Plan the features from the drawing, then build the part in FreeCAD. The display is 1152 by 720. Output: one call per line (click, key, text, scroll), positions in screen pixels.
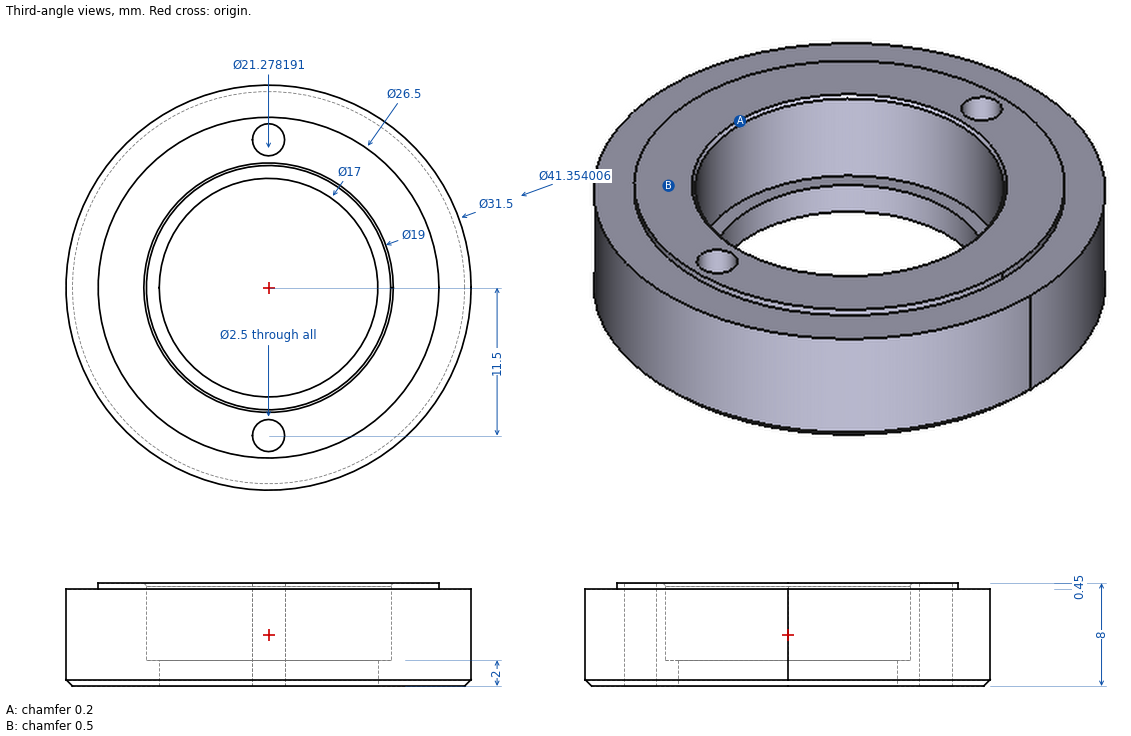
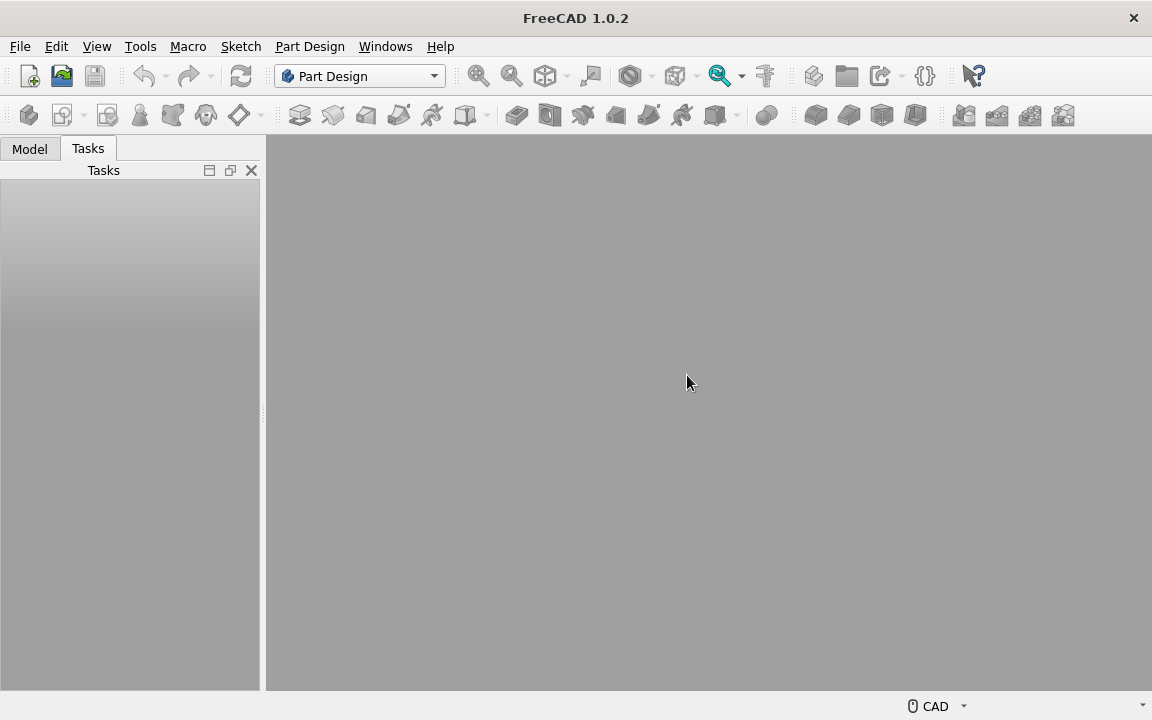
click(29, 76)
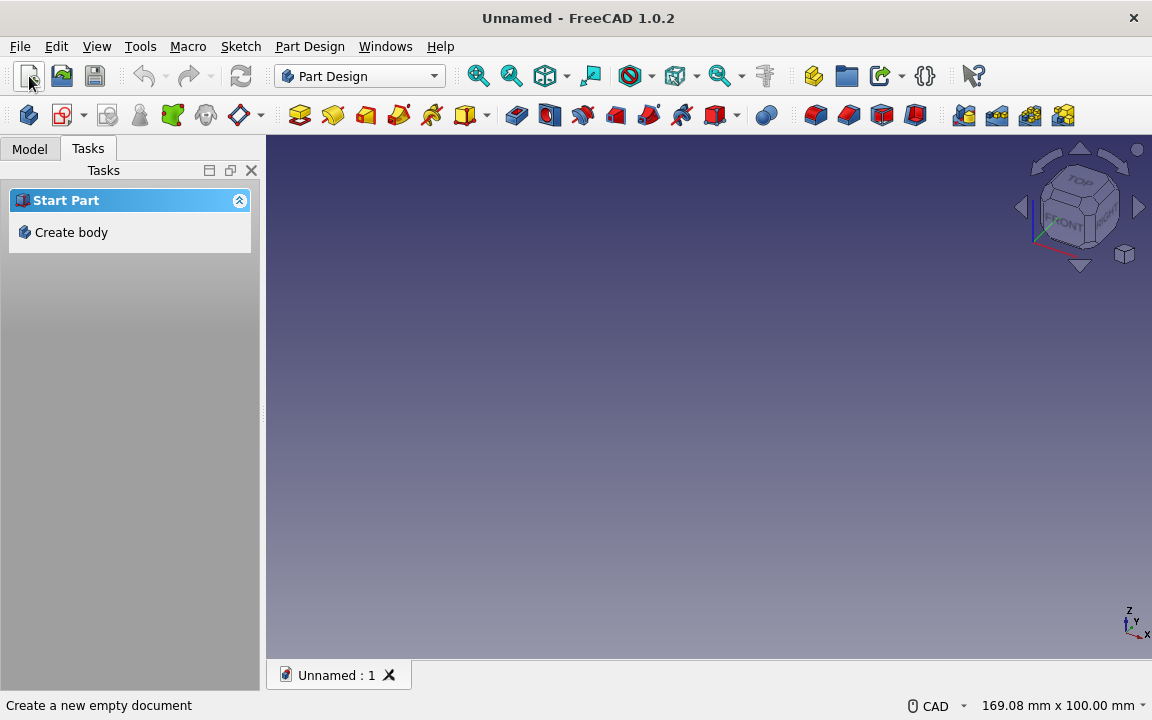
click(62, 116)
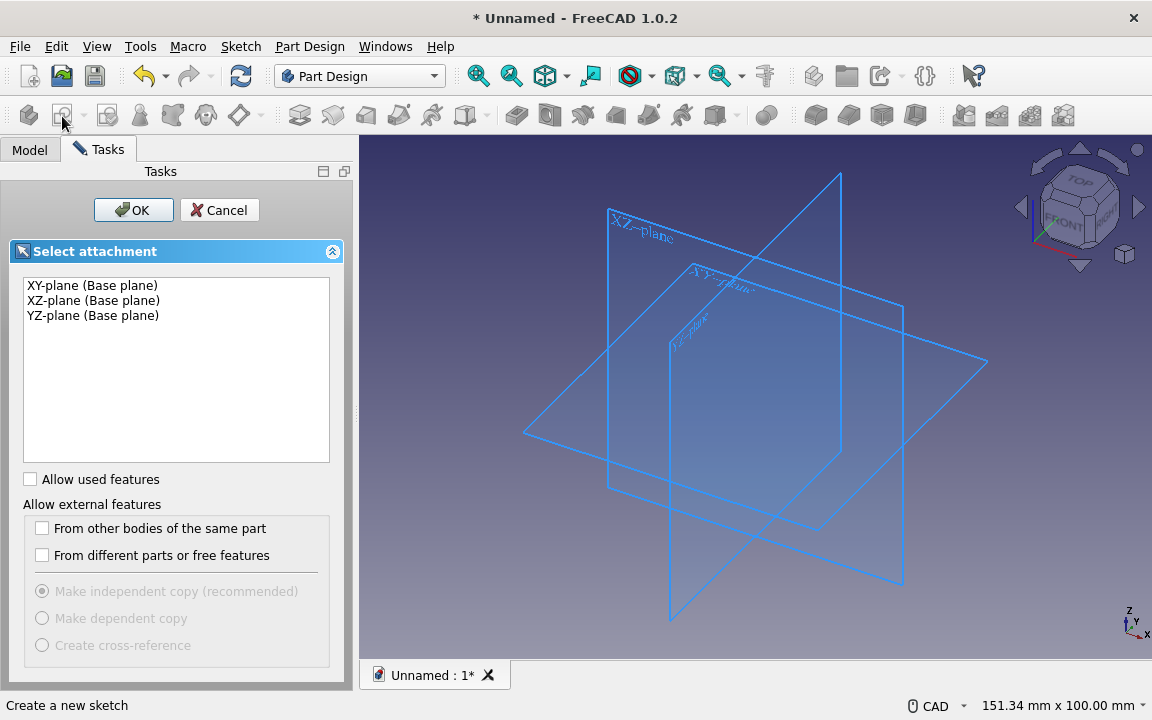
click(84, 286)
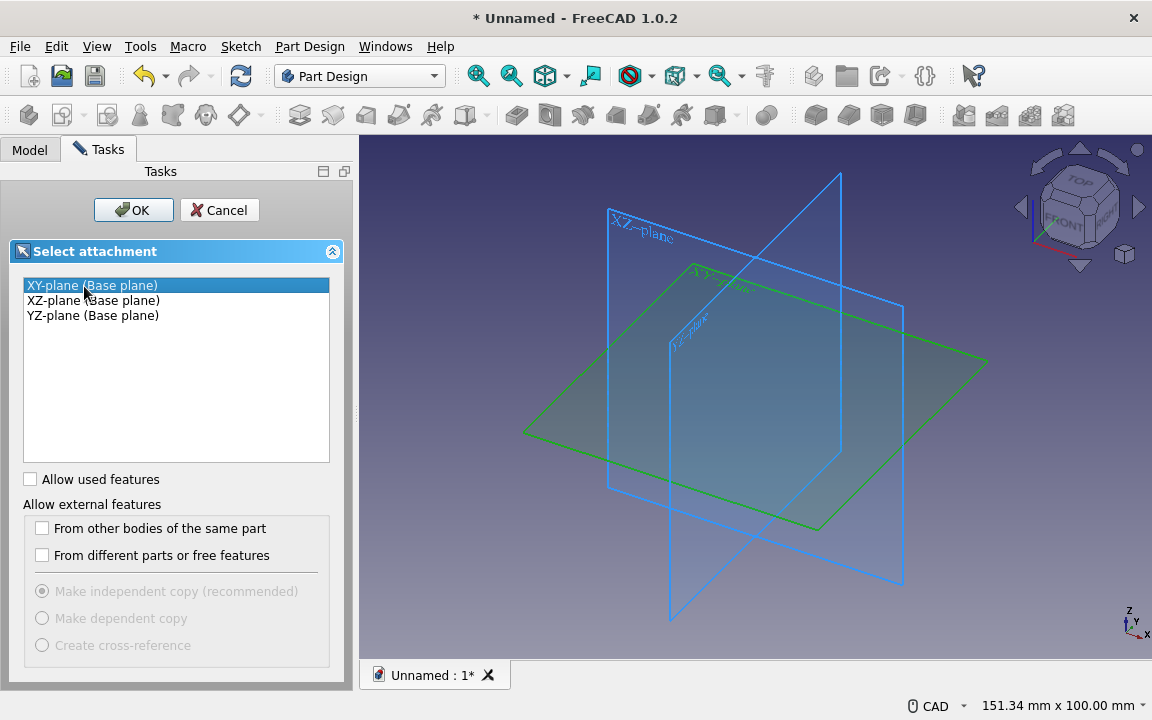
click(134, 210)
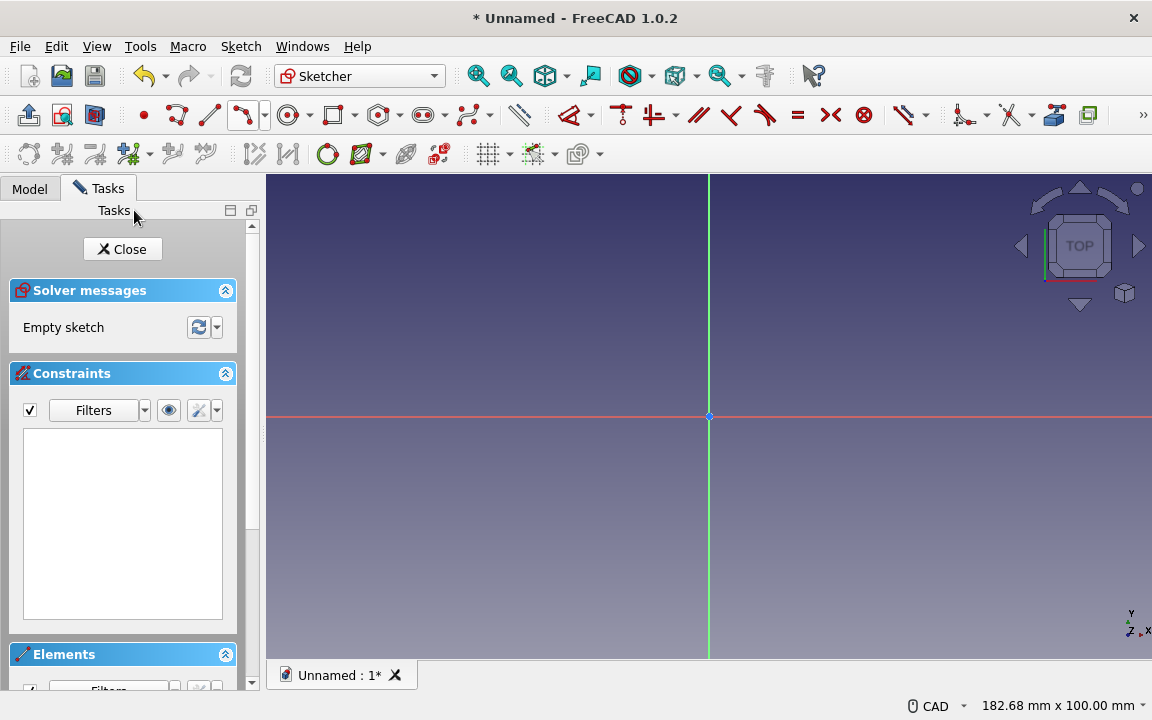
scroll(792, 416, up, 3)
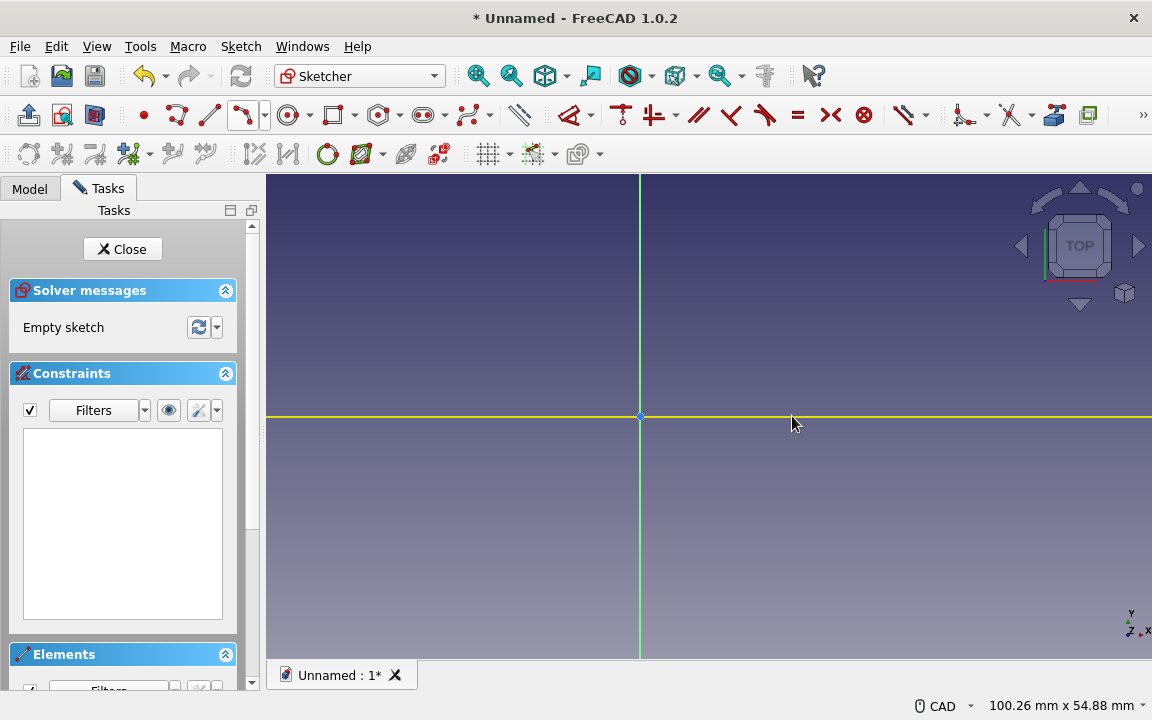
click(288, 116)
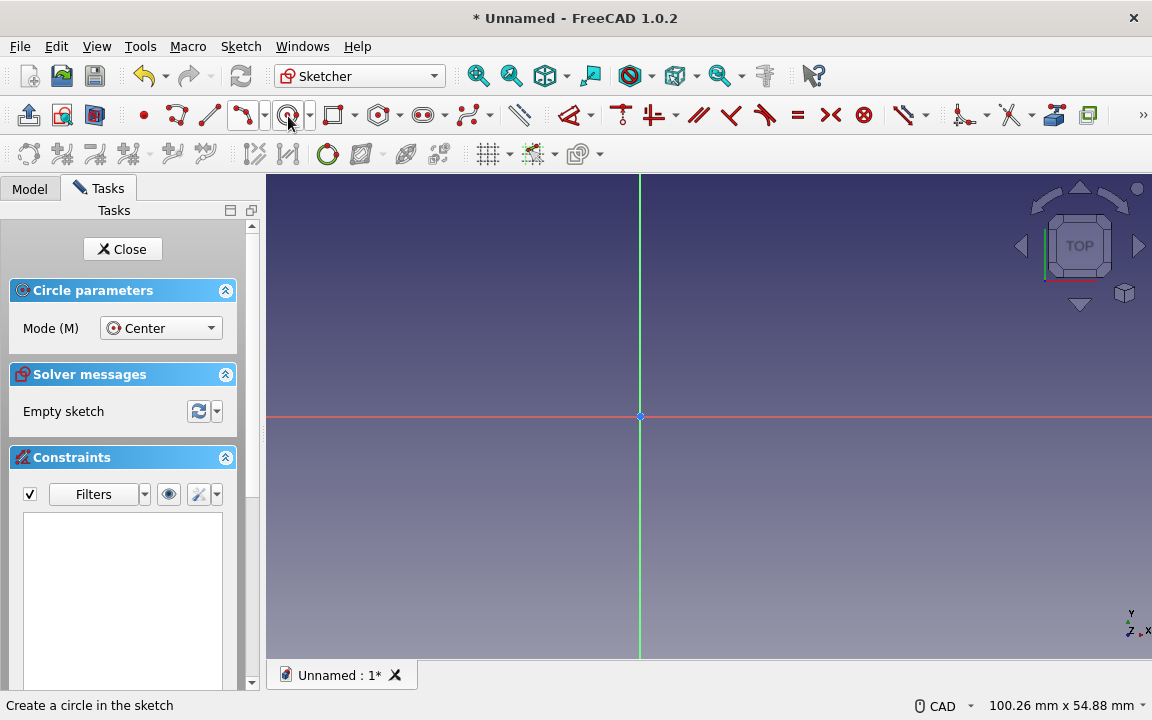
click(640, 416)
move(739, 318)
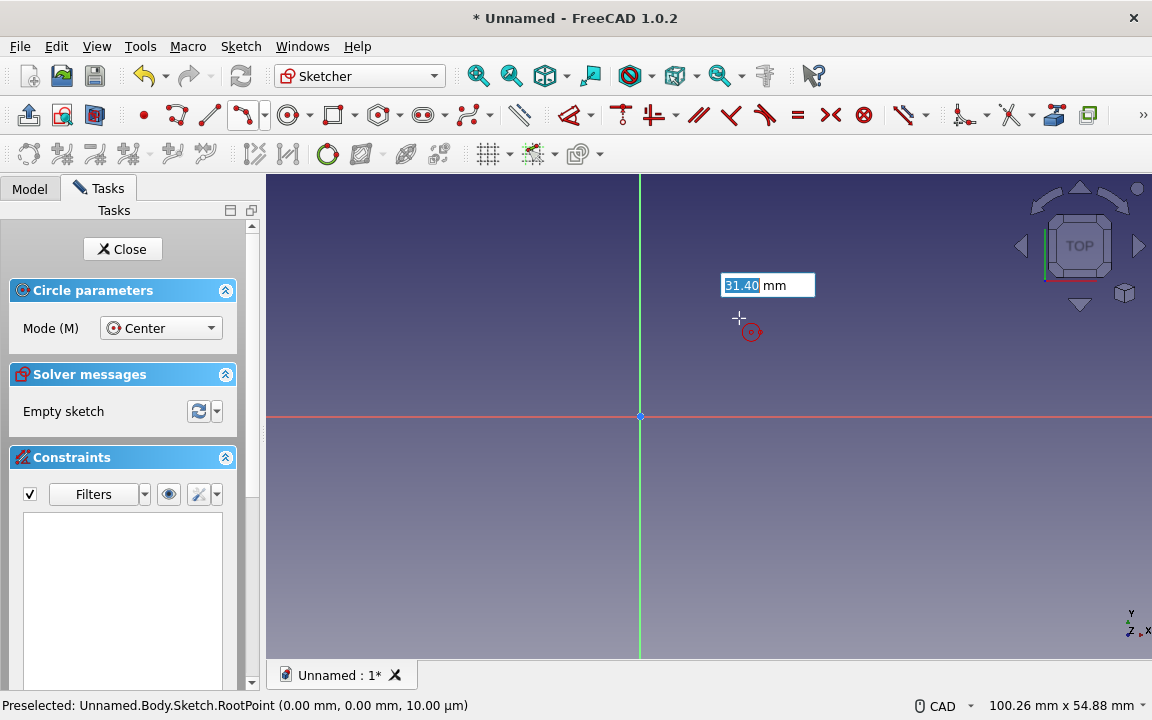
text(31.5)
key(Return)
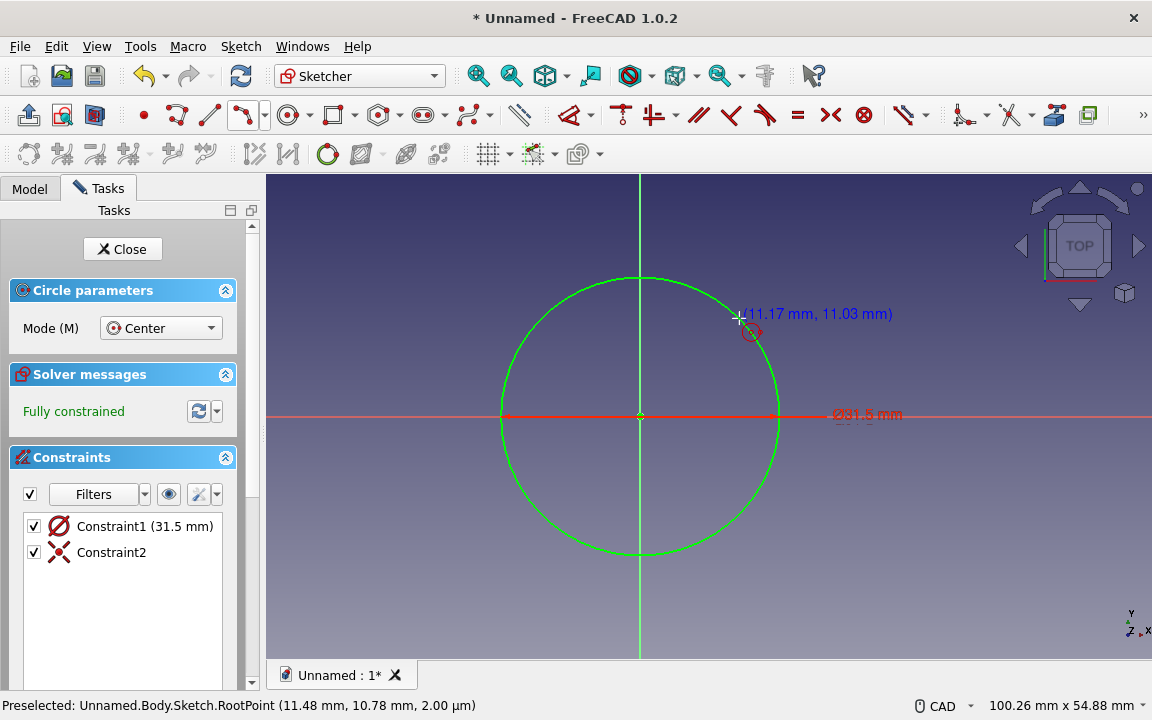
click(640, 416)
move(700, 357)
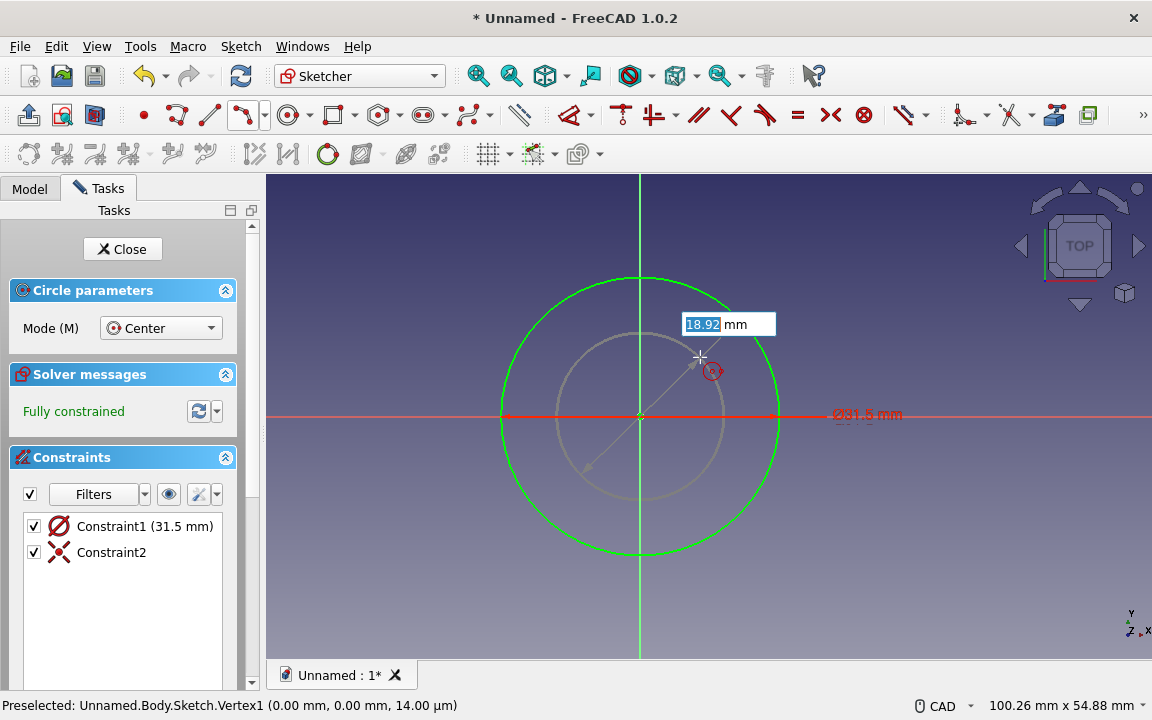
text(19)
key(Return)
key(Escape)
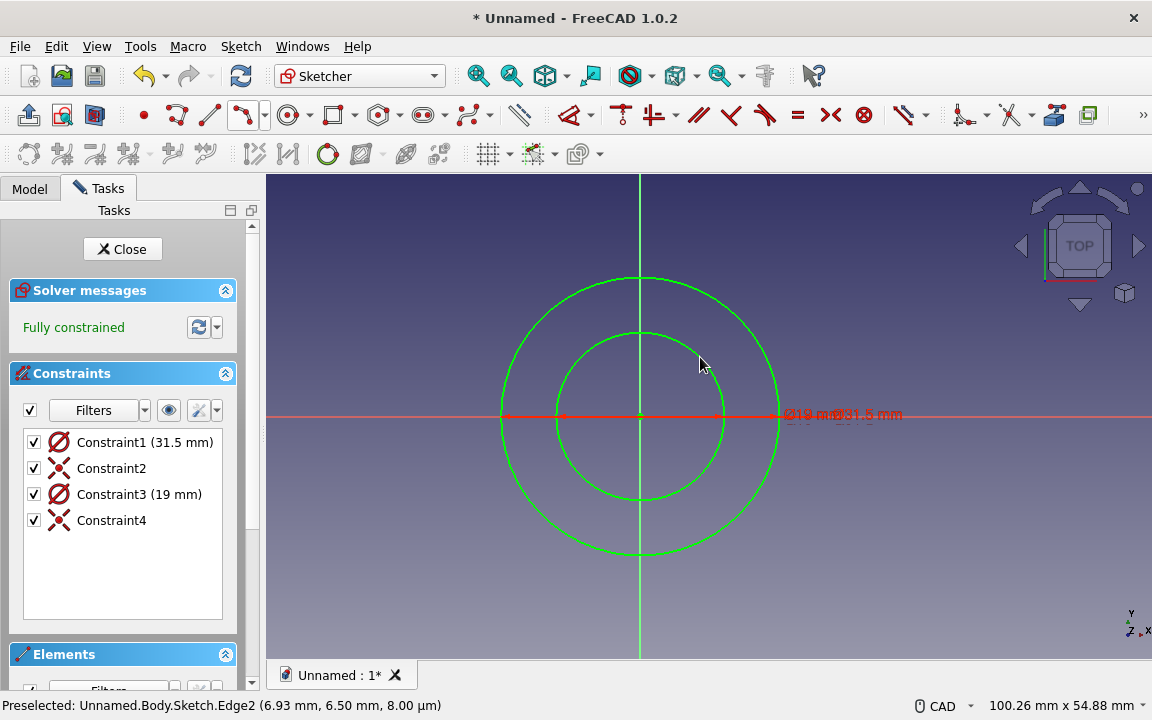
click(123, 249)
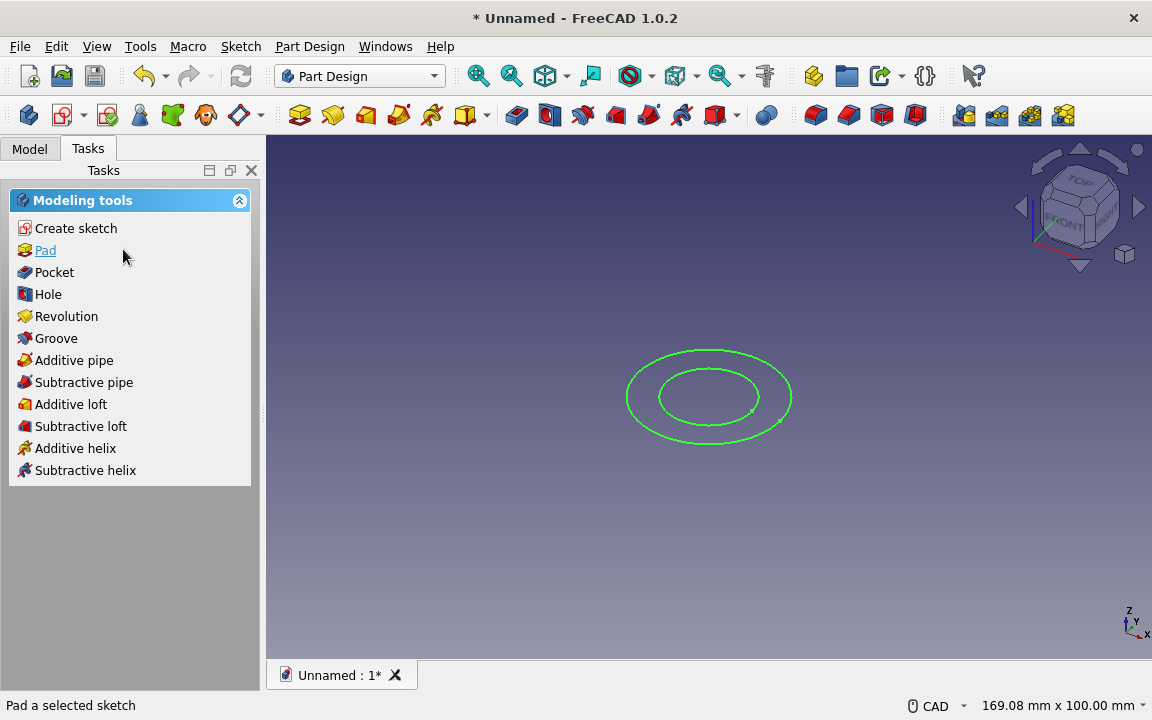
click(300, 116)